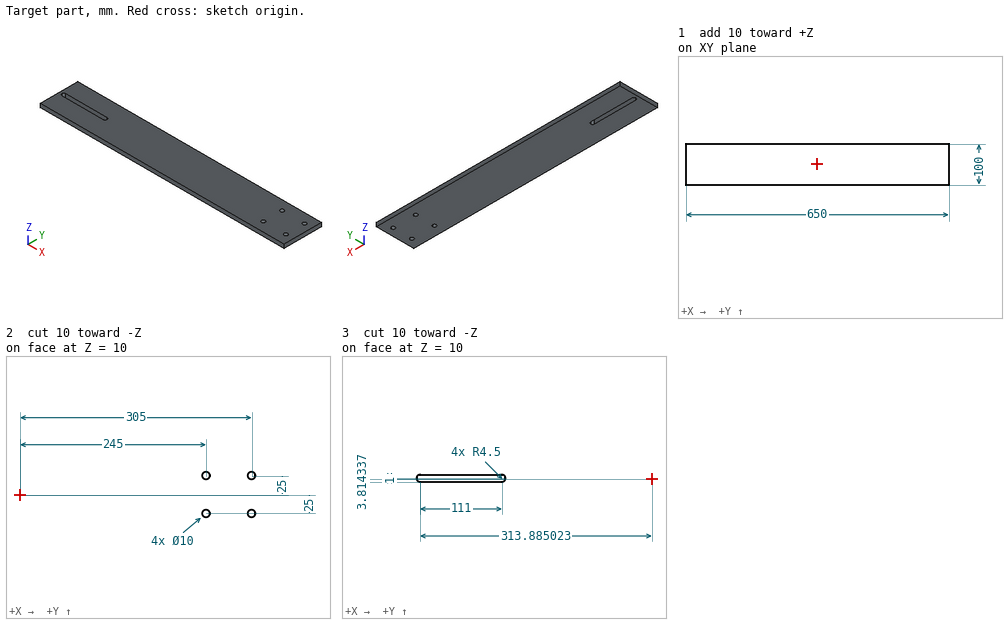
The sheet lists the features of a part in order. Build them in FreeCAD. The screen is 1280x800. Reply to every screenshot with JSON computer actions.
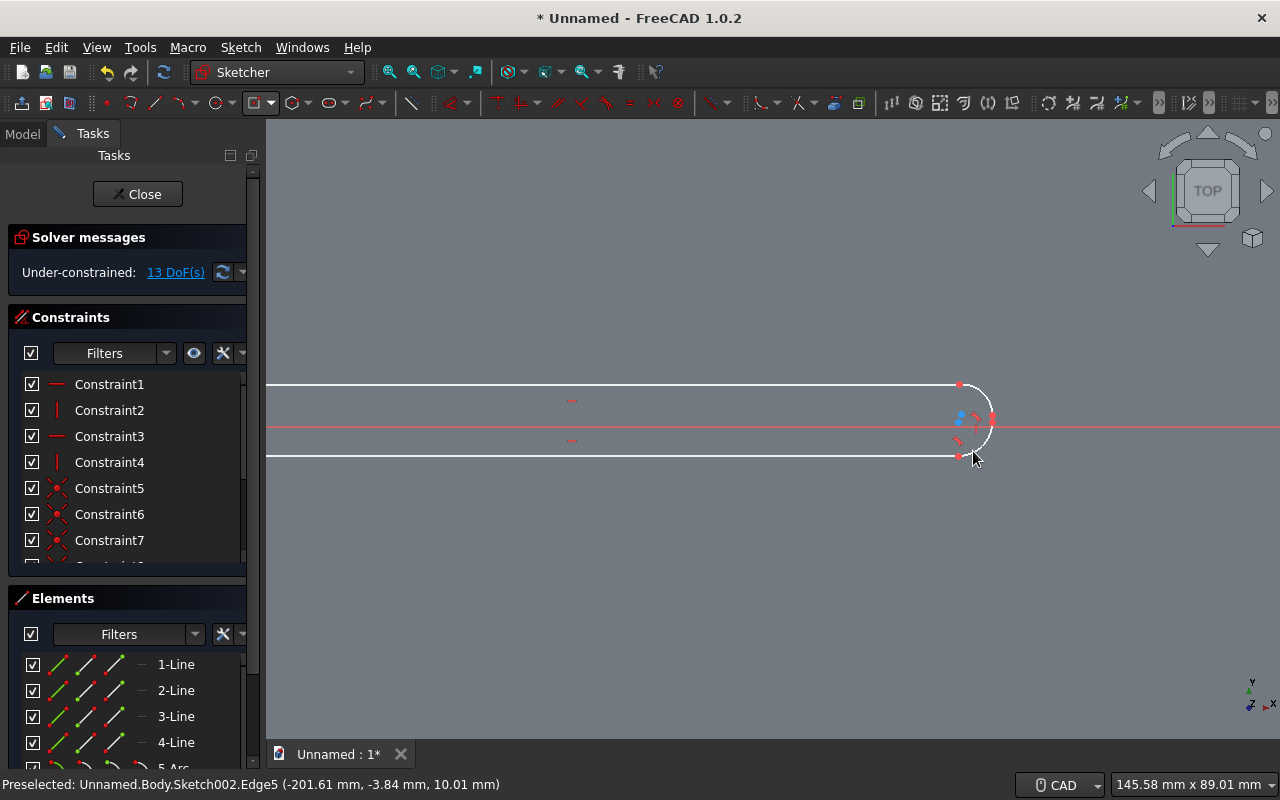
{"action": "scroll", "coordinate": [992, 419], "scroll_direction": "up", "scroll_amount": 7}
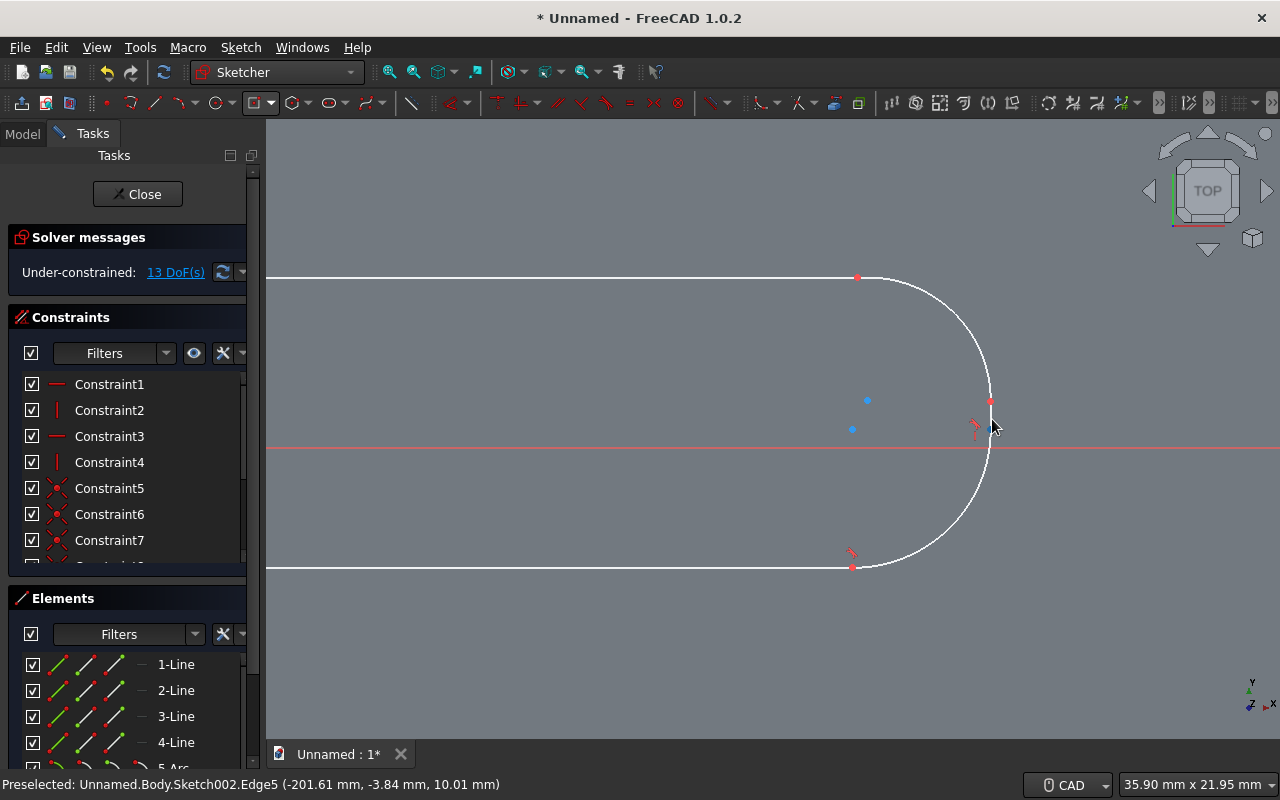
{"action": "left_click", "coordinate": [991, 416]}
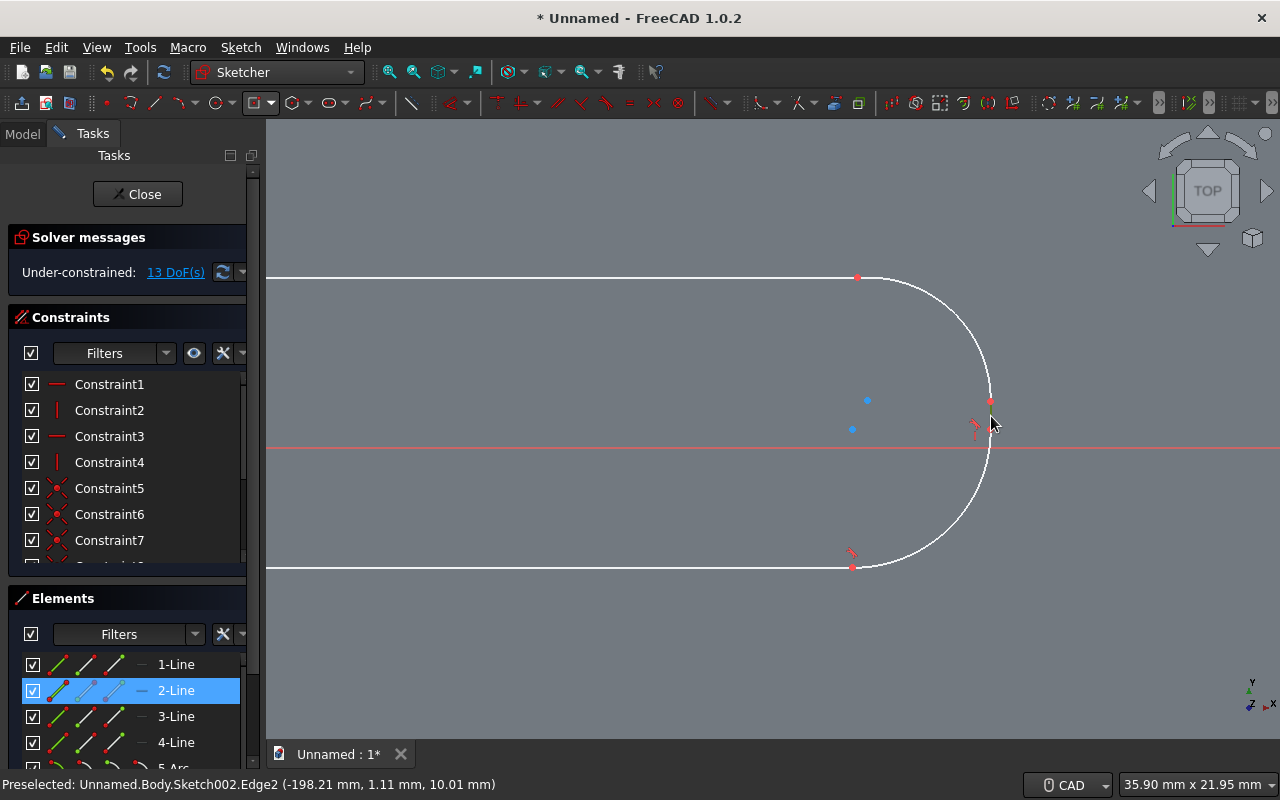
{"action": "scroll", "coordinate": [984, 432], "scroll_direction": "down", "scroll_amount": 9}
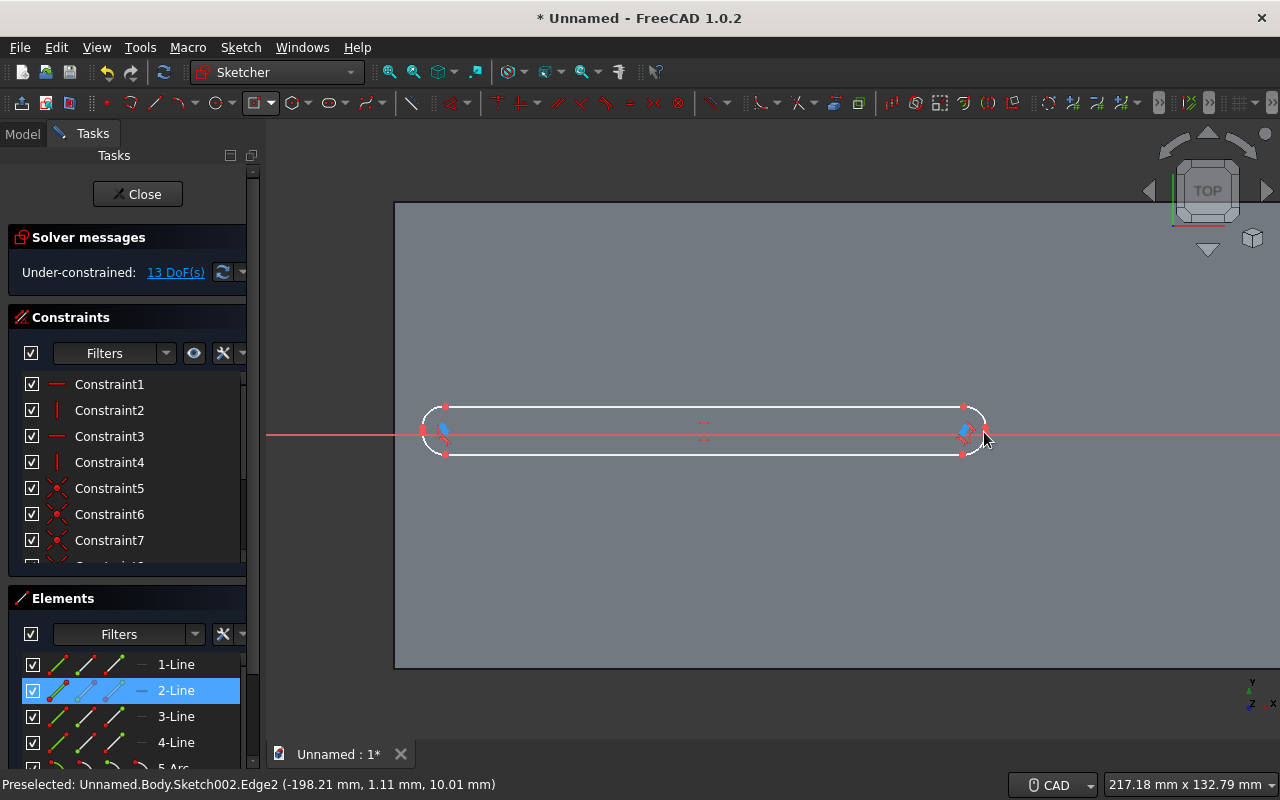
{"action": "scroll", "coordinate": [983, 418], "scroll_direction": "up", "scroll_amount": 2}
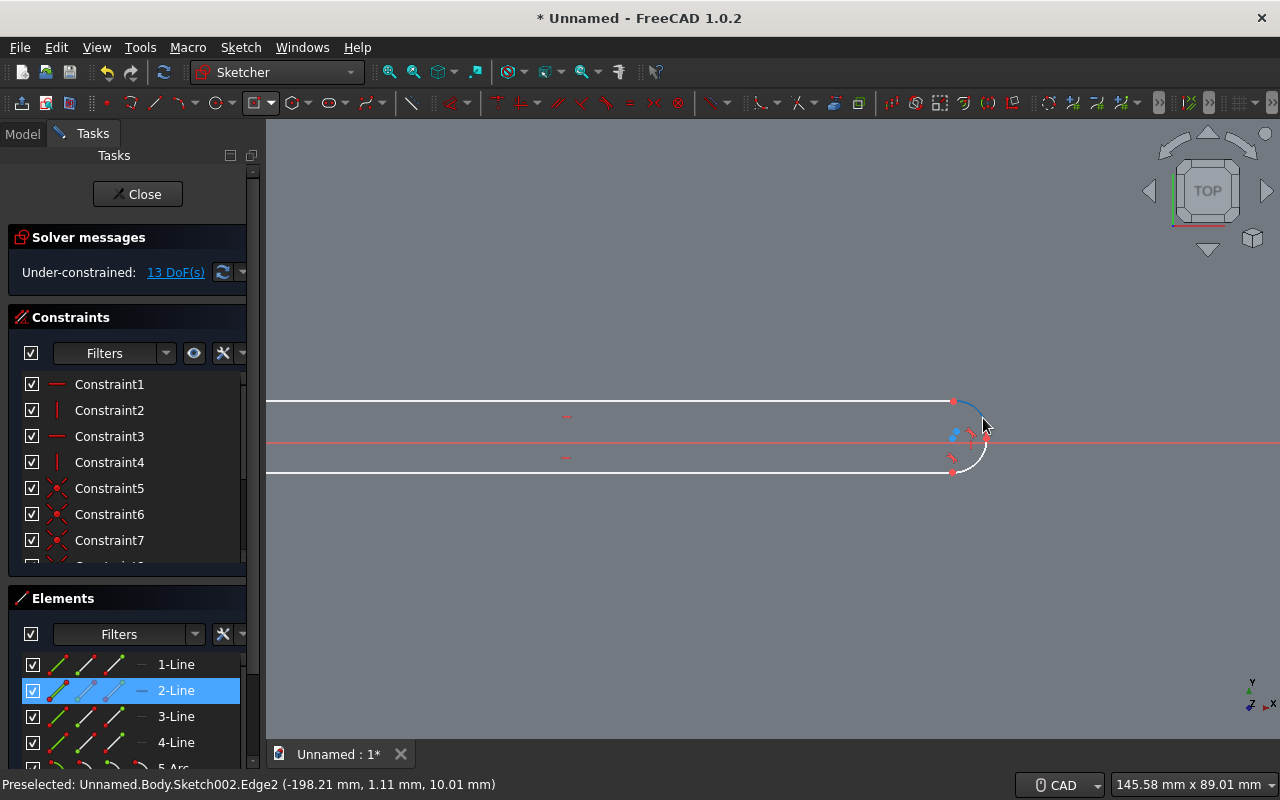
{"action": "left_click", "coordinate": [983, 417]}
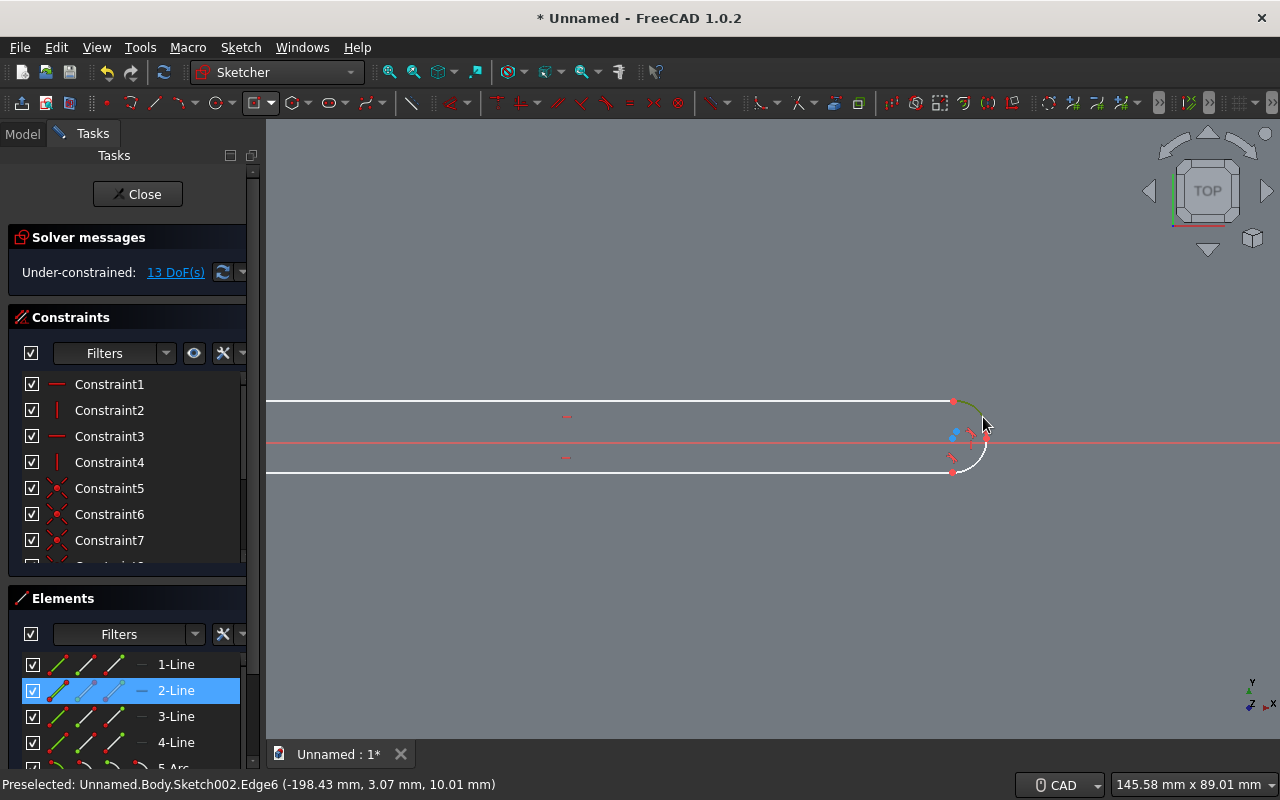
{"action": "key", "text": "t"}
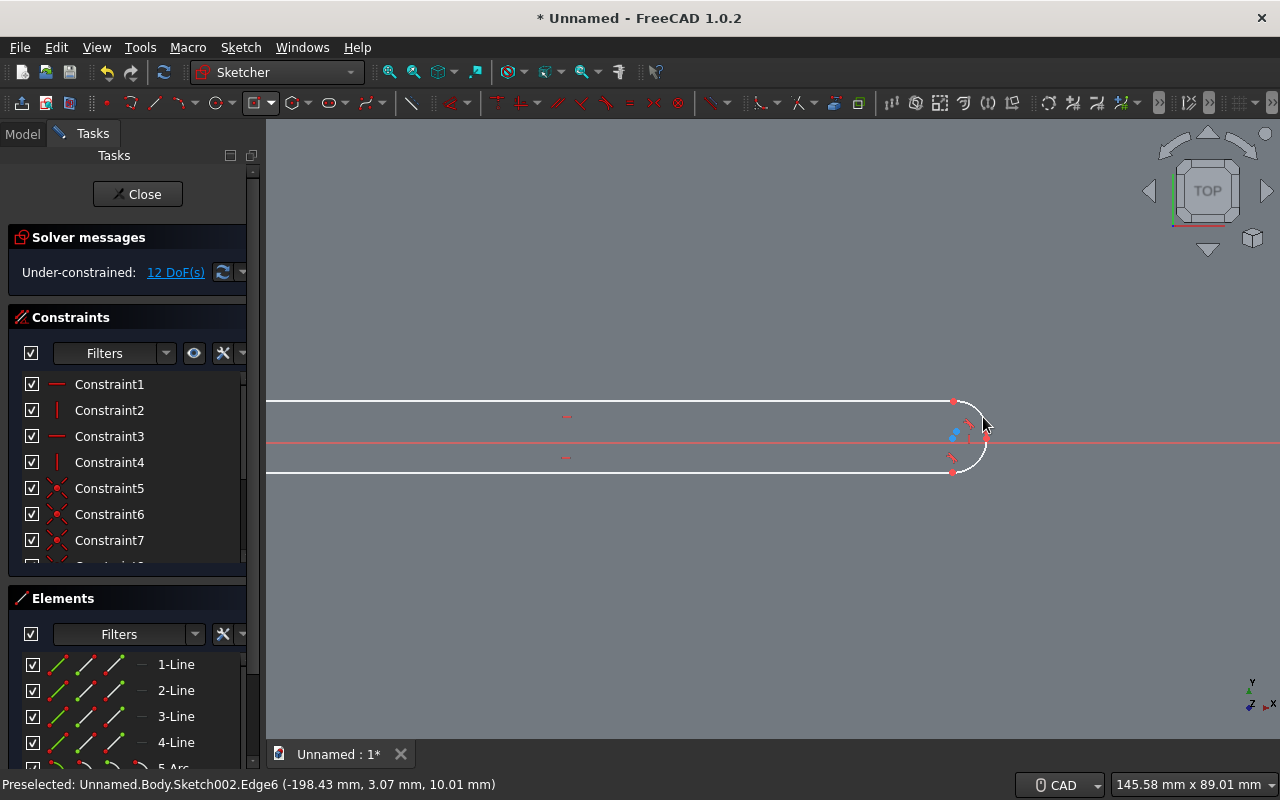
{"action": "left_click", "coordinate": [722, 401]}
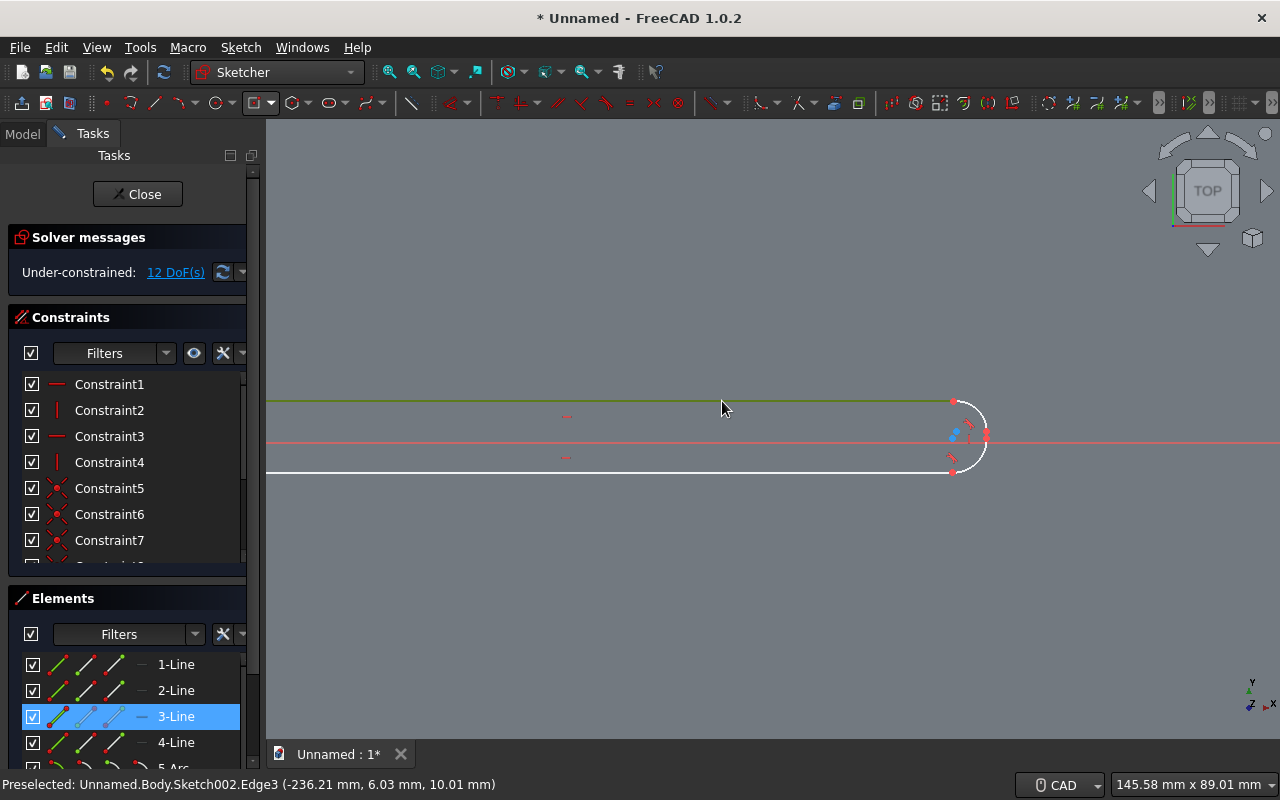
{"action": "left_click", "coordinate": [983, 417]}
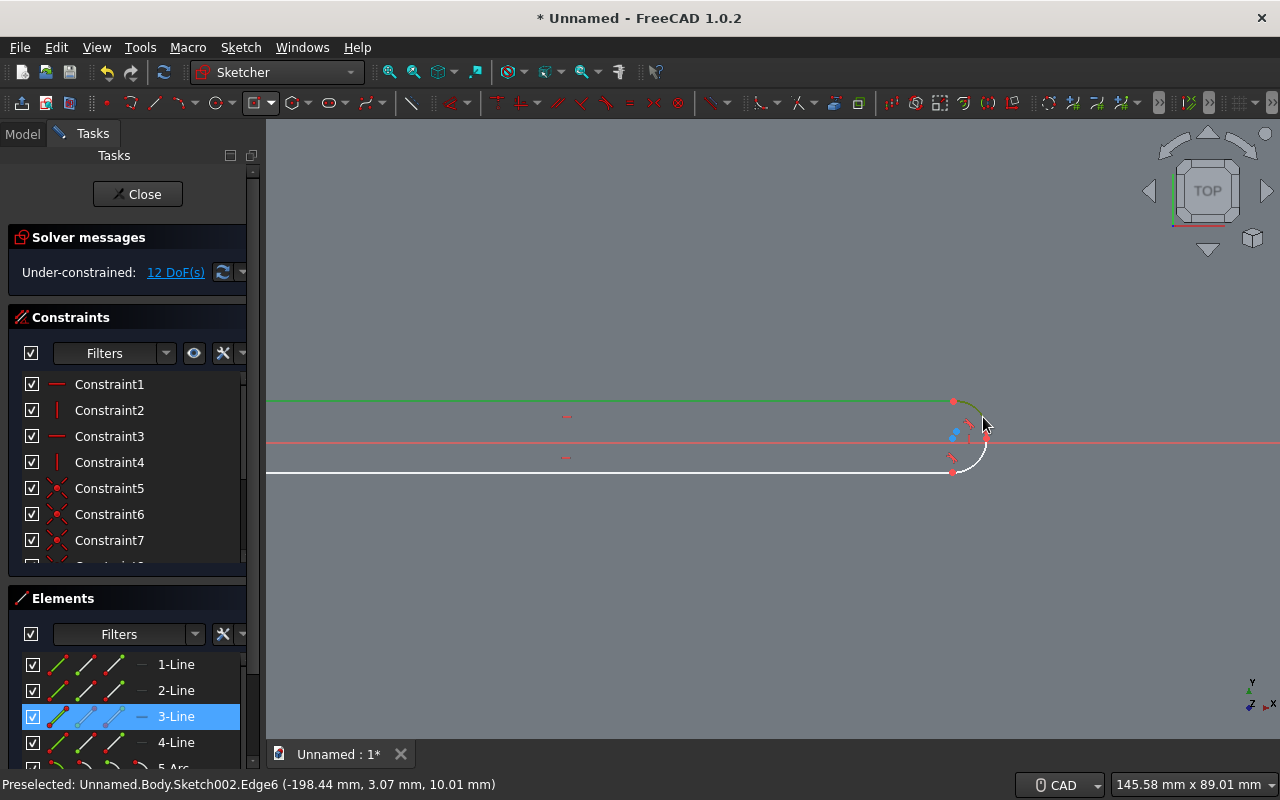
{"action": "key", "text": "t"}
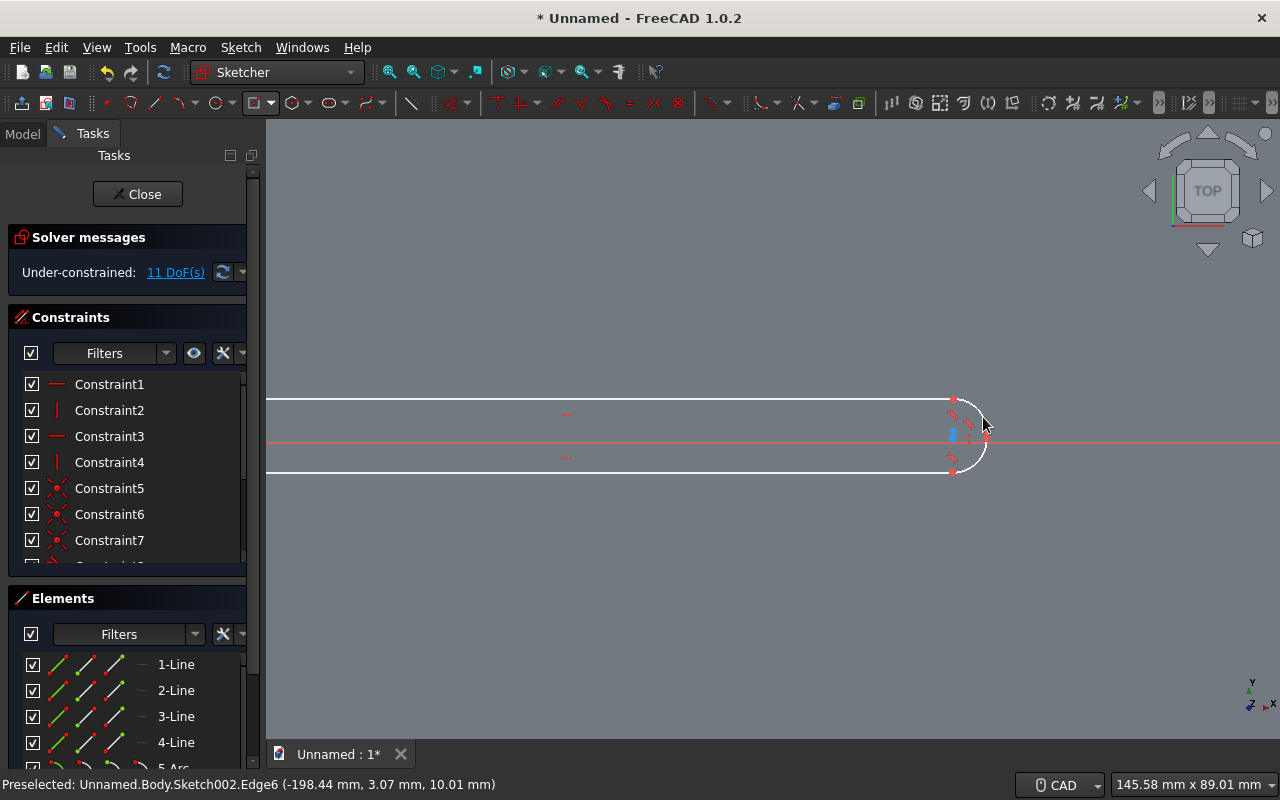
{"action": "left_click", "coordinate": [722, 399]}